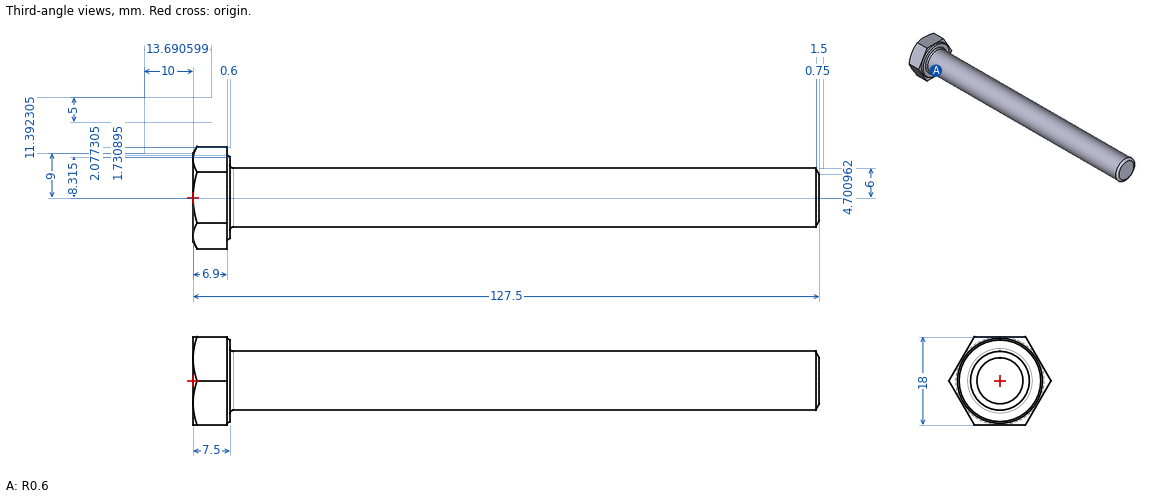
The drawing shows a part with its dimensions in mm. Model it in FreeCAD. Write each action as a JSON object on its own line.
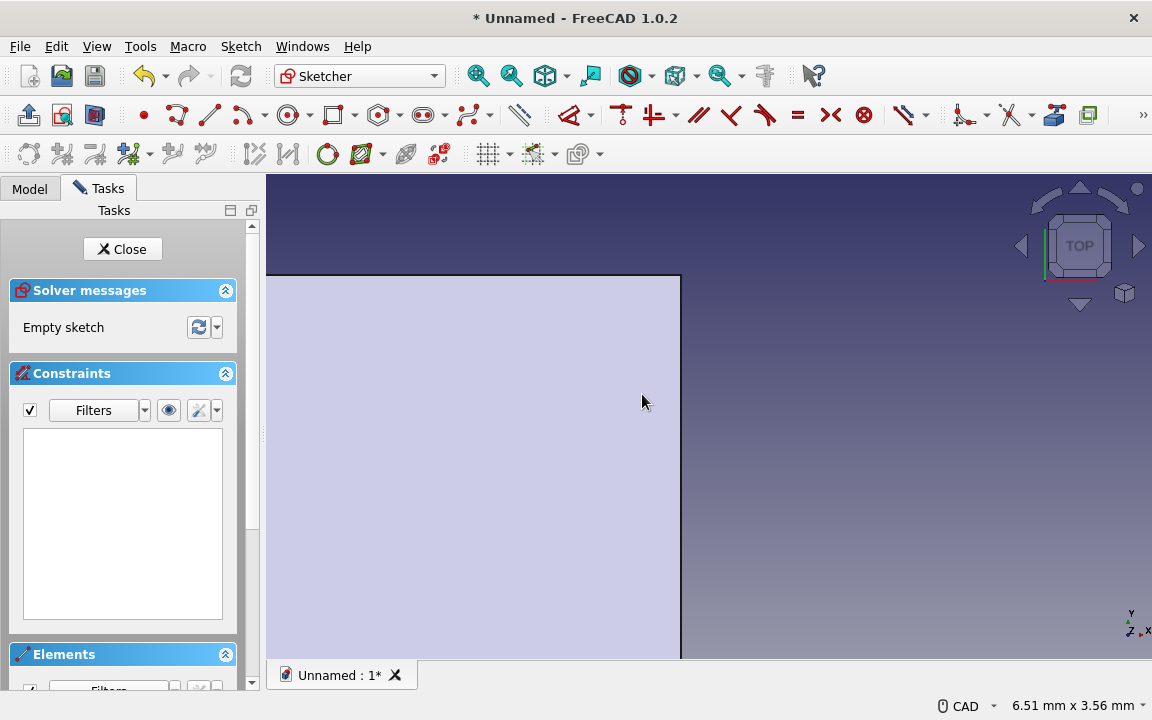
{"action": "left_click", "coordinate": [177, 116]}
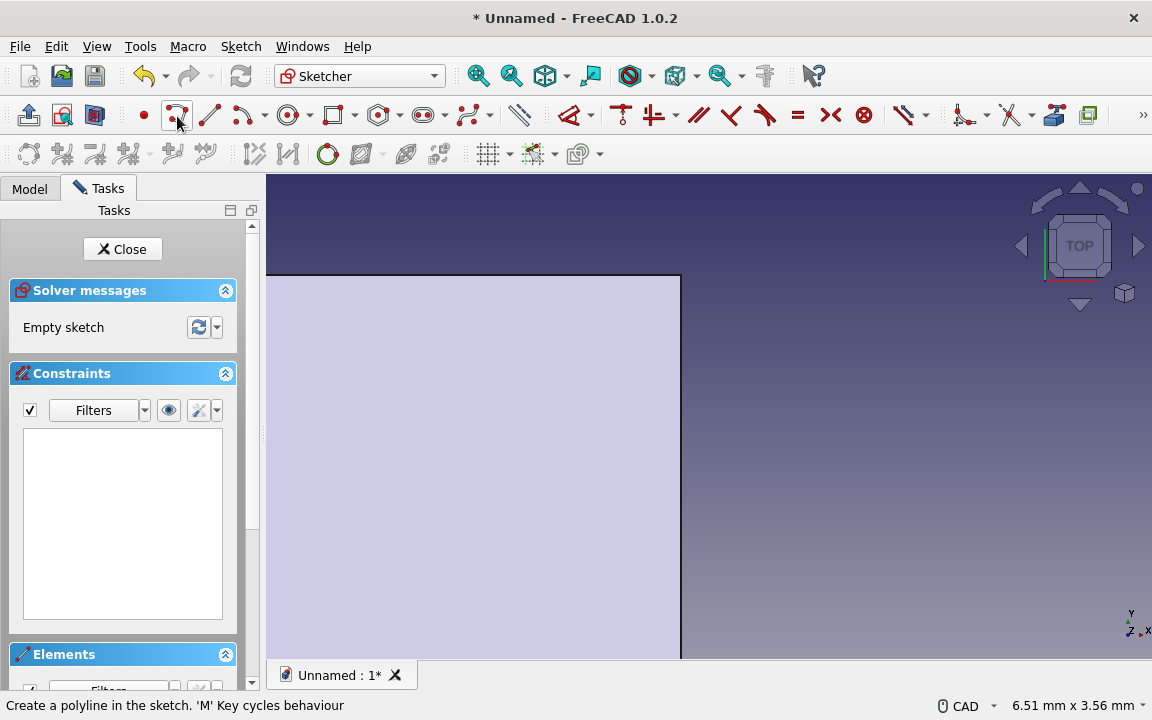
{"action": "left_click", "coordinate": [599, 510]}
{"action": "left_click", "coordinate": [681, 558]}
{"action": "left_click", "coordinate": [681, 275]}
{"action": "left_click", "coordinate": [599, 275]}
{"action": "left_click", "coordinate": [599, 511]}
{"action": "key", "text": "Escape"}
{"action": "key", "text": "Escape"}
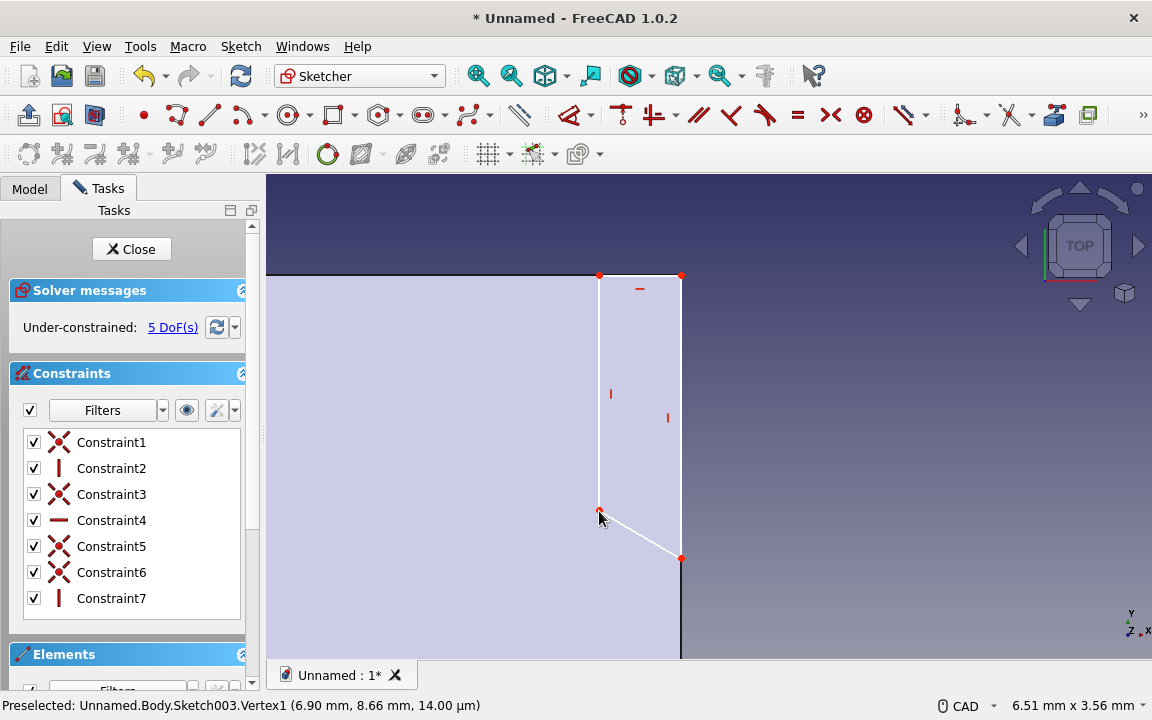
{"action": "left_click", "coordinate": [568, 116]}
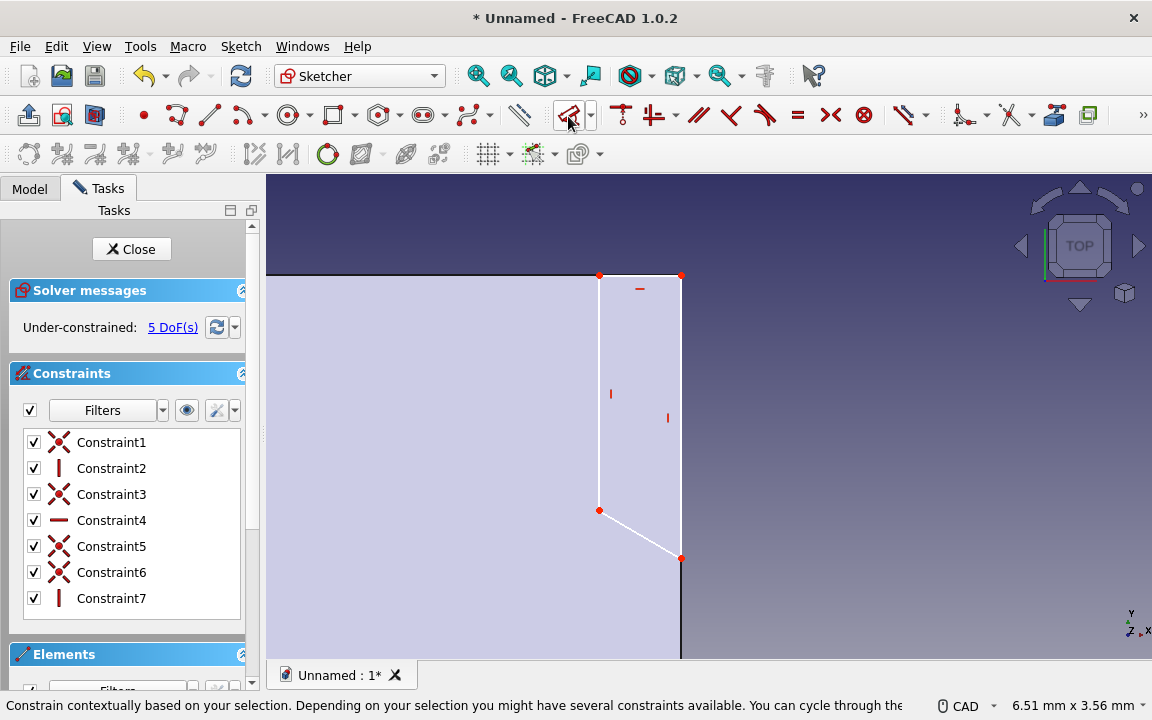
{"action": "left_click", "coordinate": [656, 276]}
{"action": "left_click", "coordinate": [640, 242]}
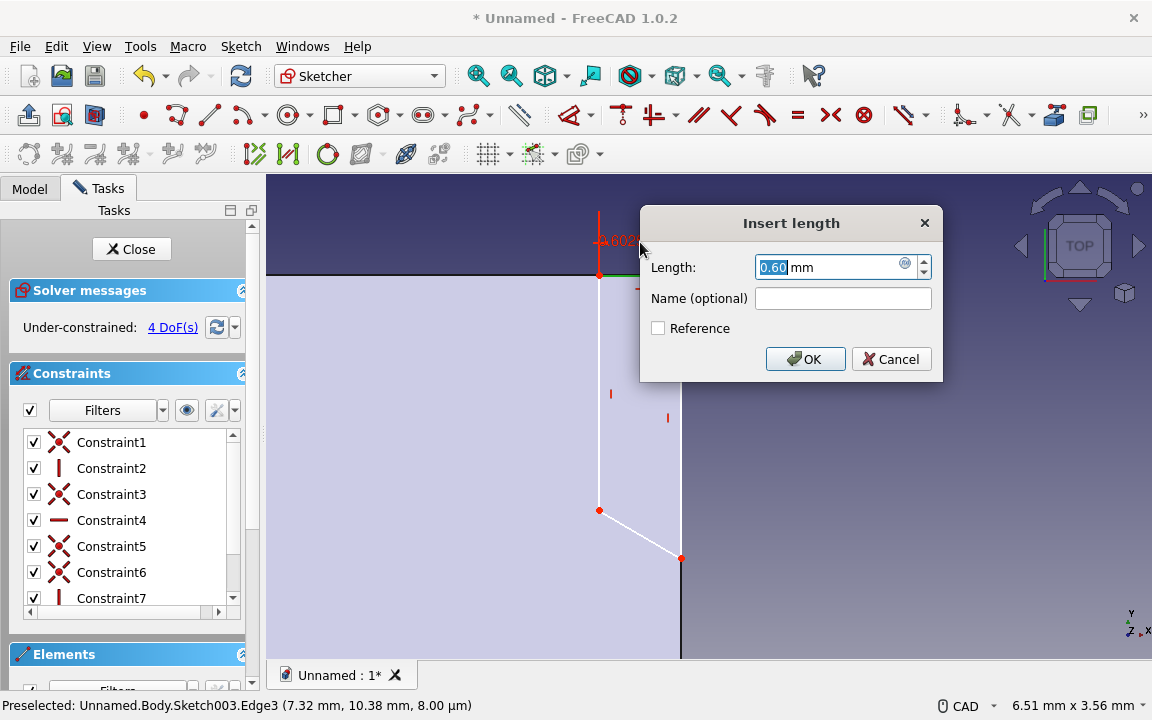
{"action": "type", "text": "0.6"}
{"action": "key", "text": "Return"}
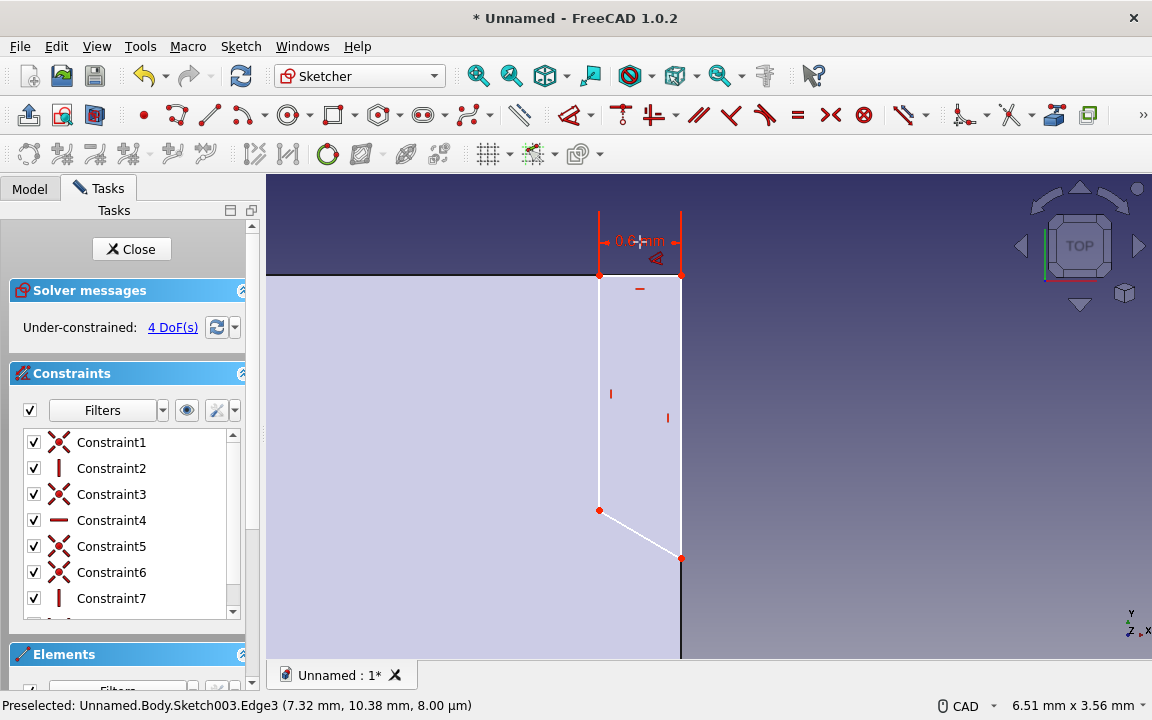
{"action": "left_click", "coordinate": [599, 511]}
{"action": "left_click", "coordinate": [447, 477]}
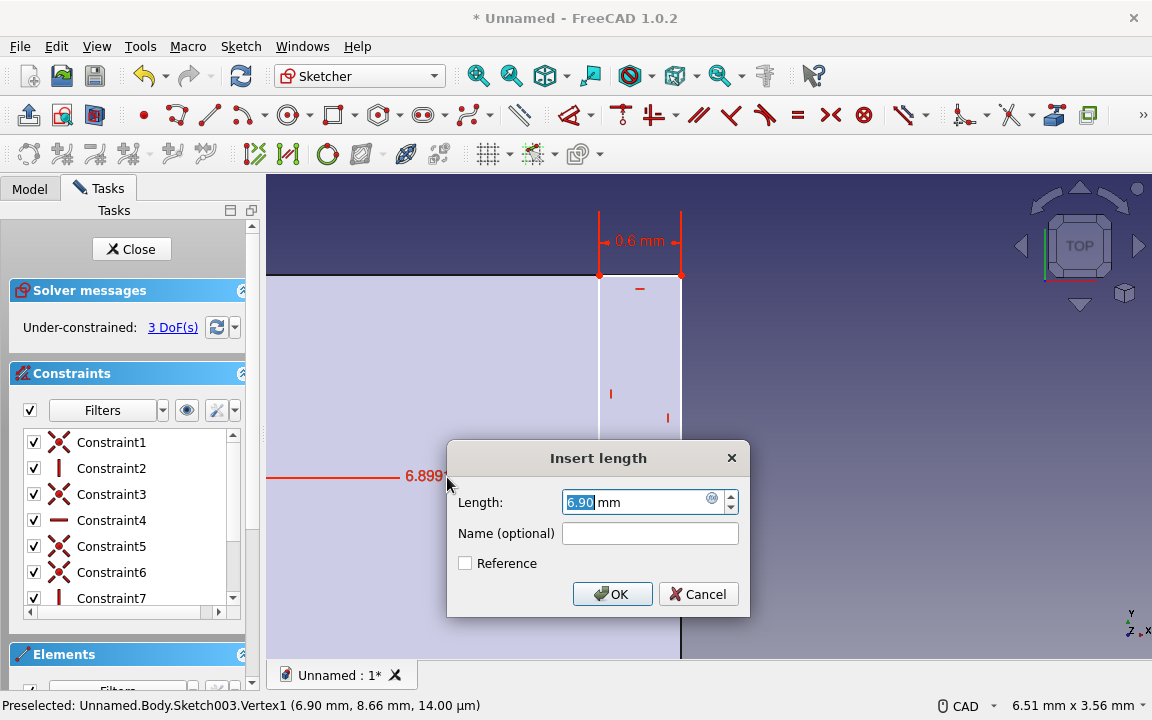
{"action": "type", "text": "6.9"}
{"action": "key", "text": "Return"}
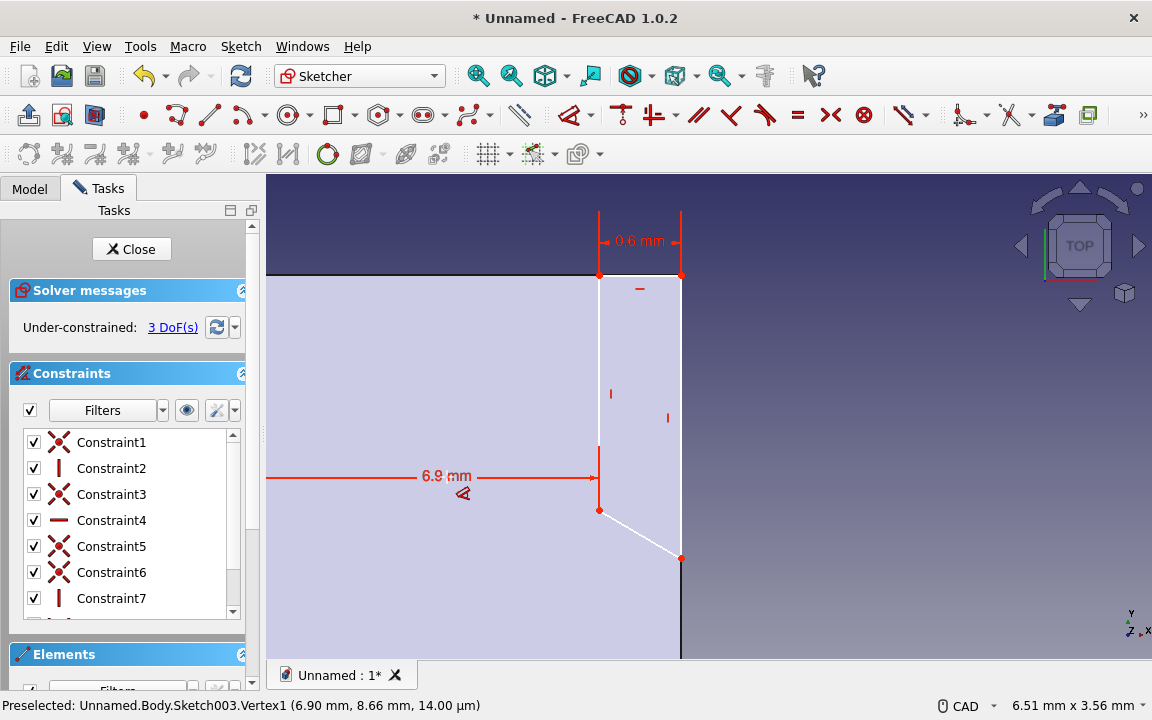
{"action": "left_click", "coordinate": [681, 559]}
{"action": "left_click", "coordinate": [715, 595]}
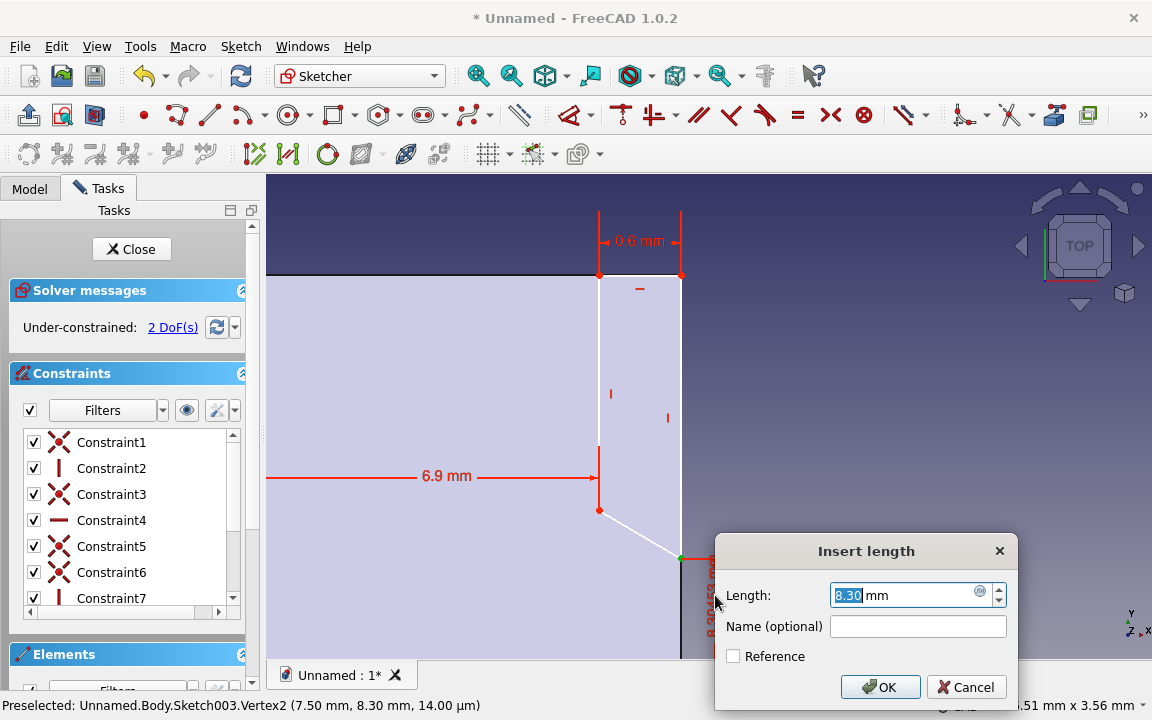
{"action": "type", "text": "8.315"}
{"action": "key", "text": "Return"}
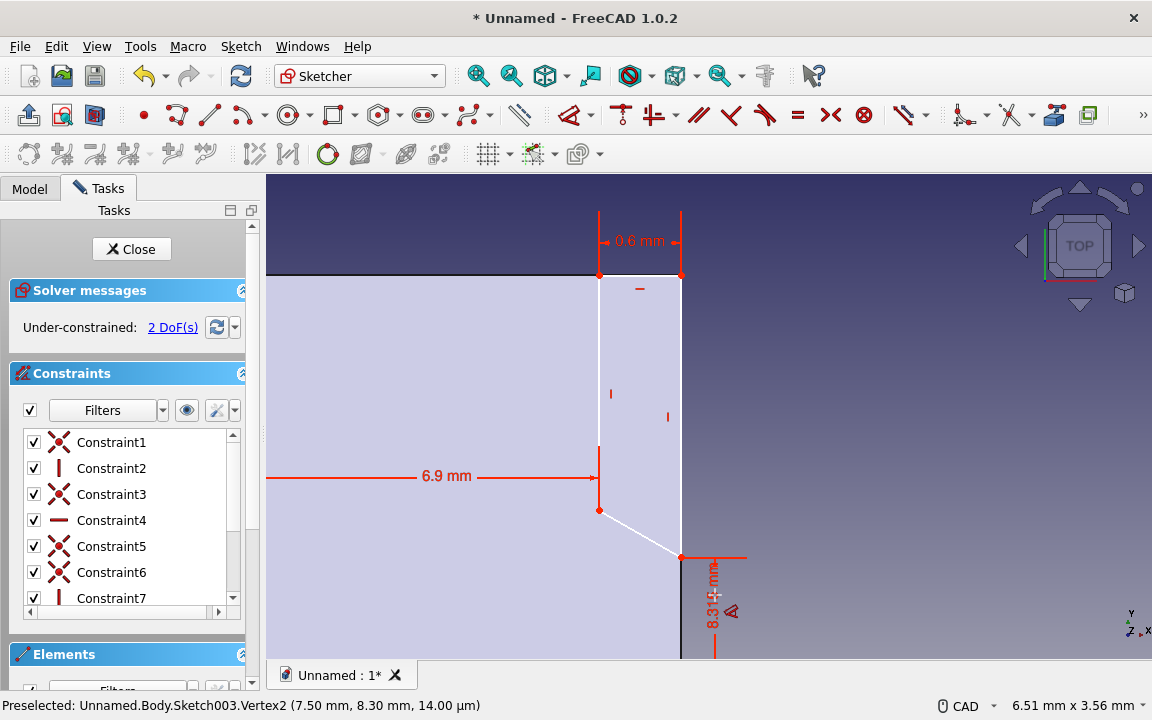
{"action": "left_click", "coordinate": [681, 473]}
{"action": "left_click", "coordinate": [715, 417]}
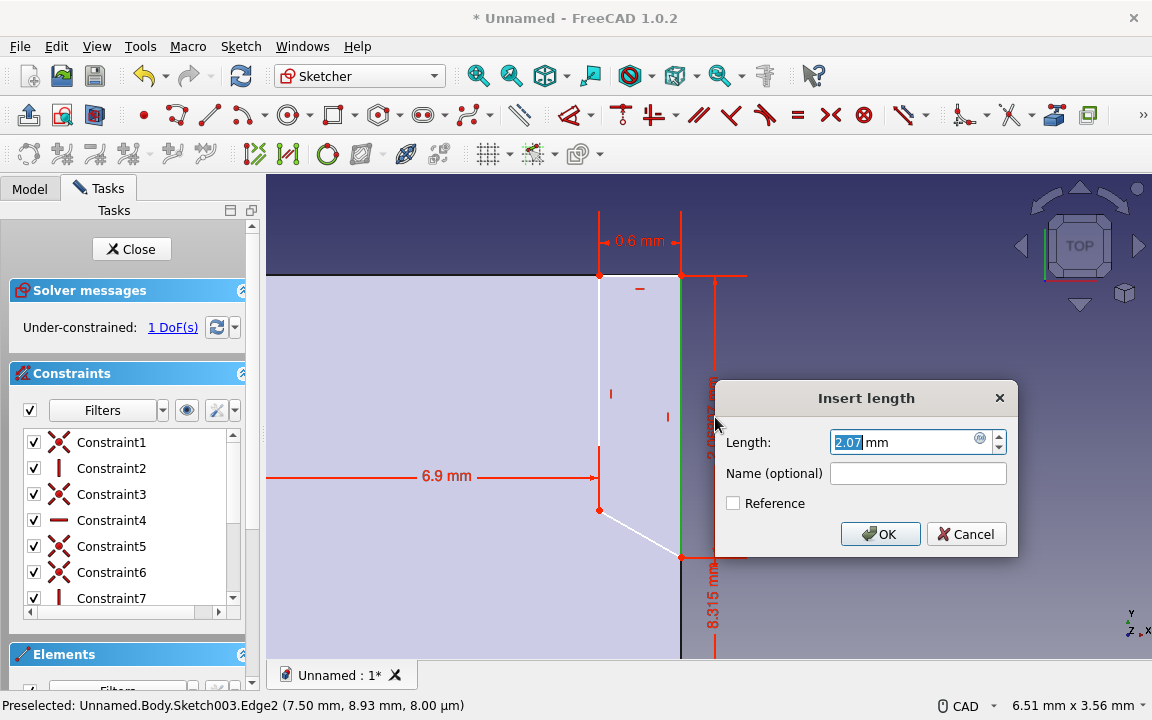
{"action": "type", "text": "2.077305"}
{"action": "key", "text": "Return"}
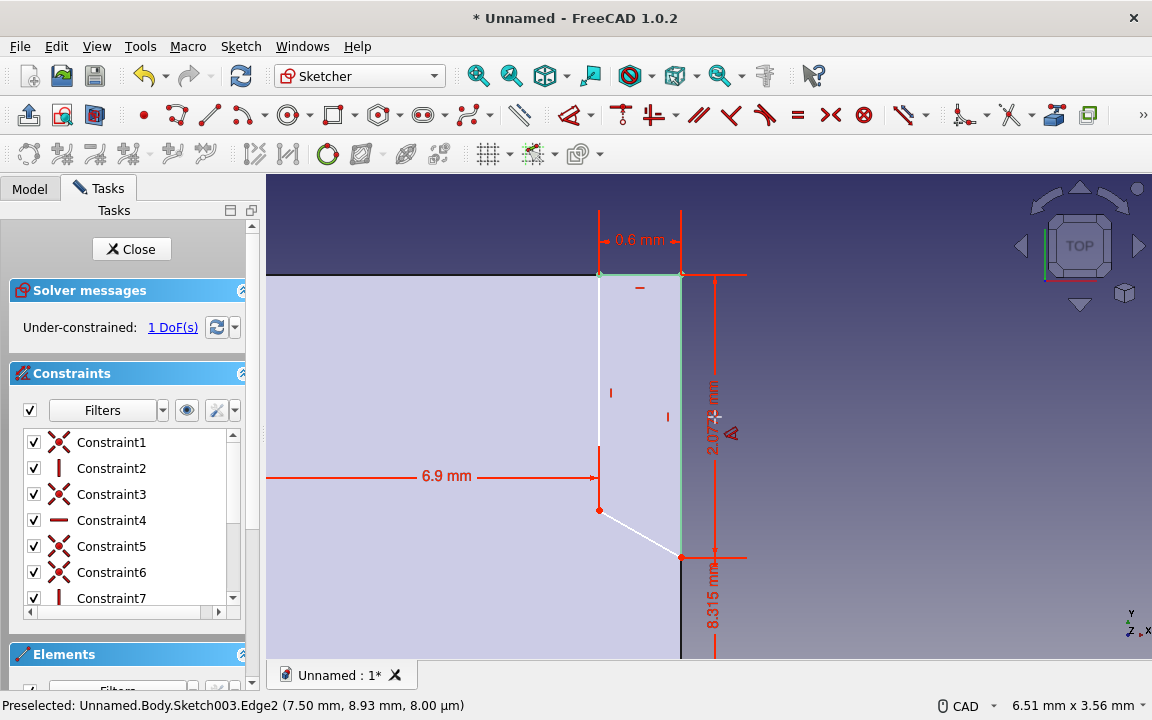
{"action": "left_click", "coordinate": [599, 346]}
{"action": "left_click", "coordinate": [565, 393]}